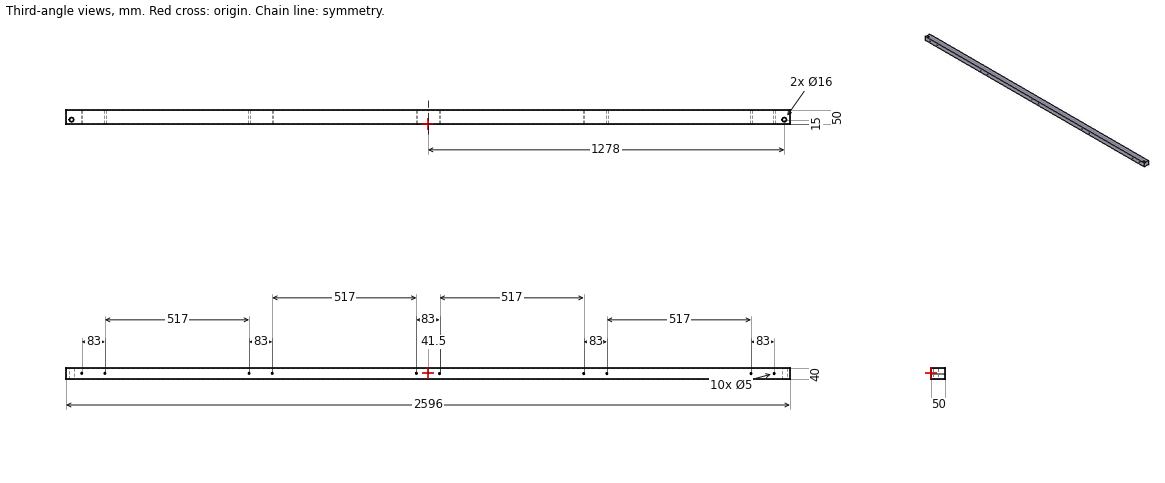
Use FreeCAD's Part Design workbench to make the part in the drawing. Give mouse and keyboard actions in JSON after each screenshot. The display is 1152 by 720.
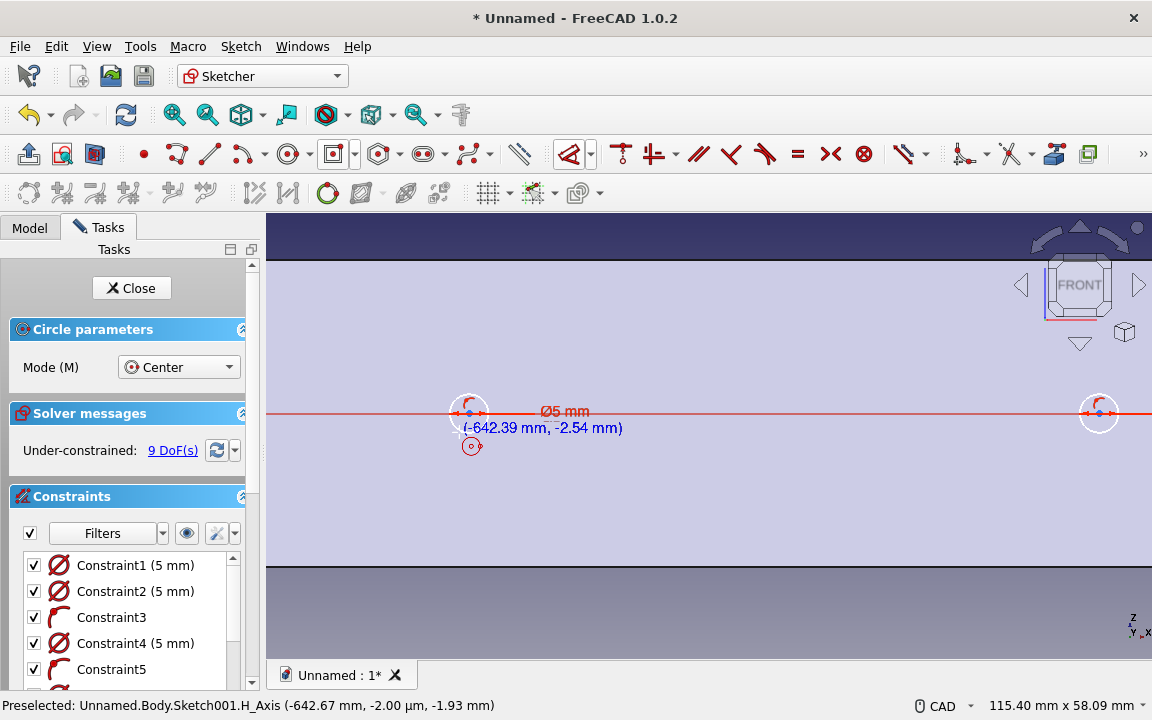
{"action": "scroll", "coordinate": [476, 437], "scroll_direction": "down", "scroll_amount": 17}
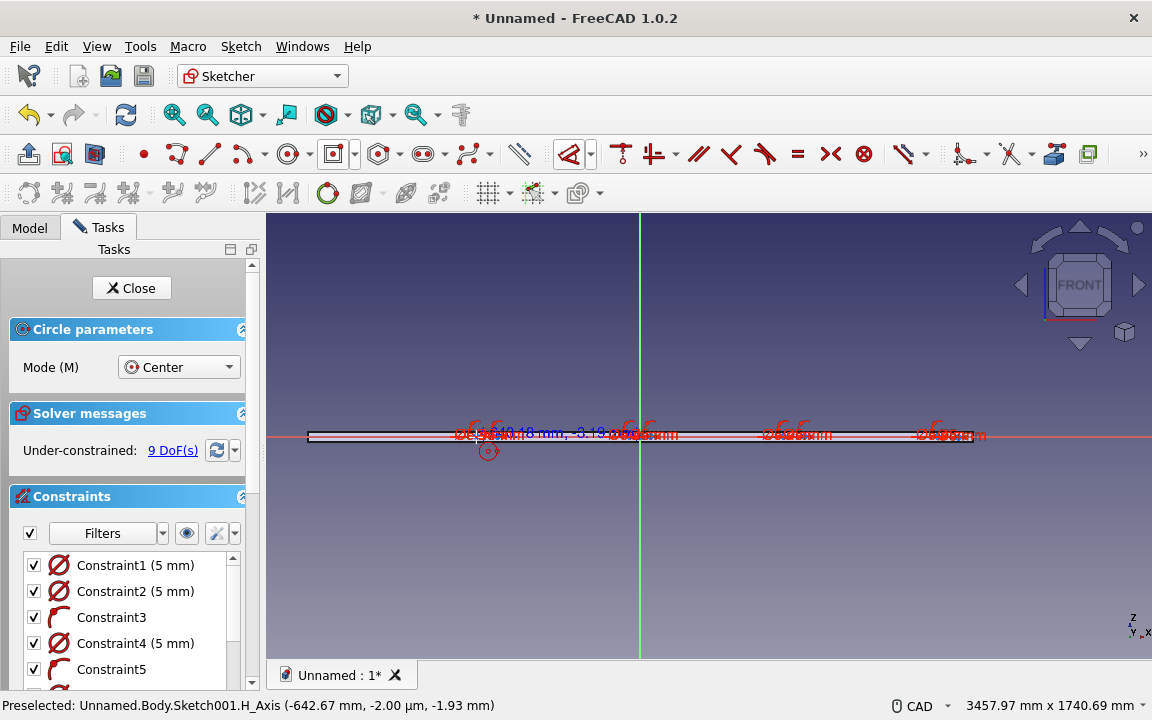
{"action": "scroll", "coordinate": [343, 437], "scroll_direction": "up", "scroll_amount": 18}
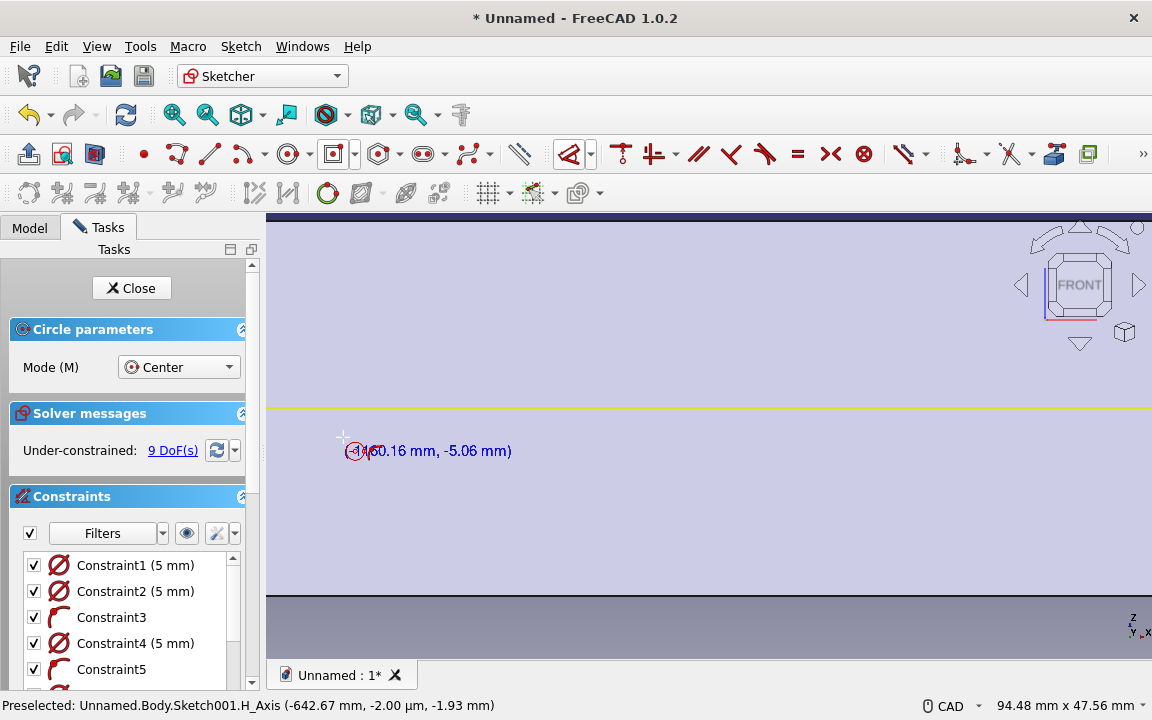
{"action": "scroll", "coordinate": [343, 437], "scroll_direction": "down", "scroll_amount": 18}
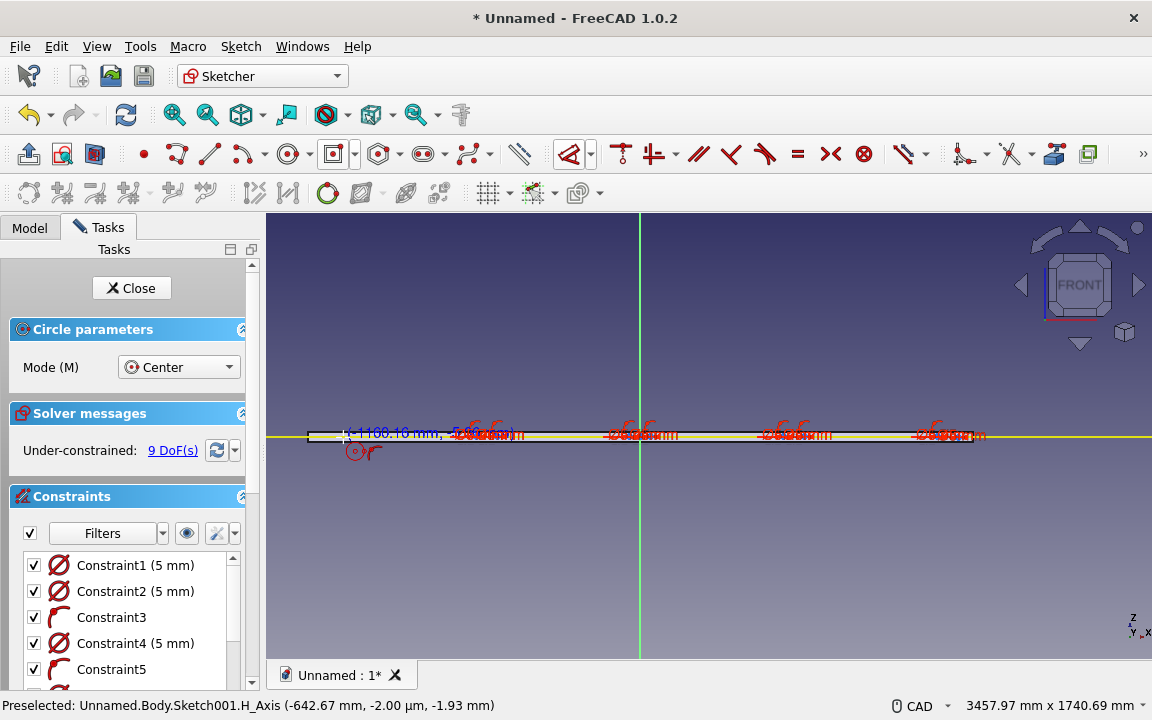
{"action": "left_click", "coordinate": [343, 437]}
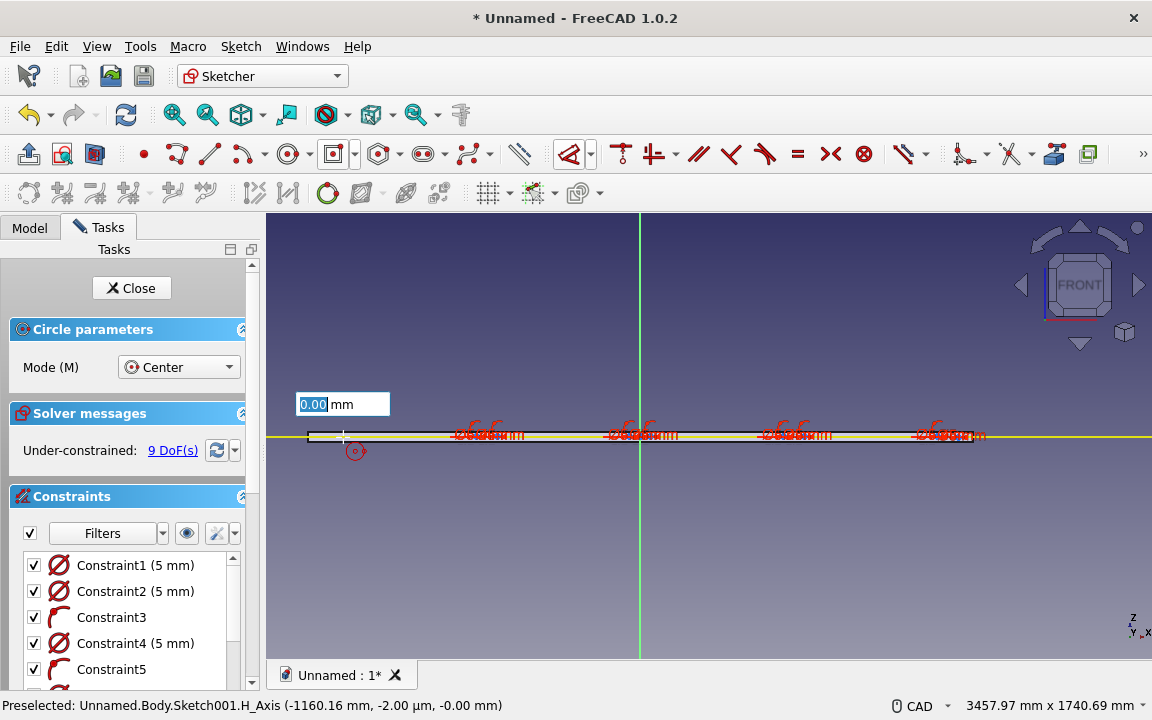
{"action": "scroll", "coordinate": [343, 437], "scroll_direction": "up", "scroll_amount": 17}
{"action": "mouse_move", "coordinate": [347, 432]}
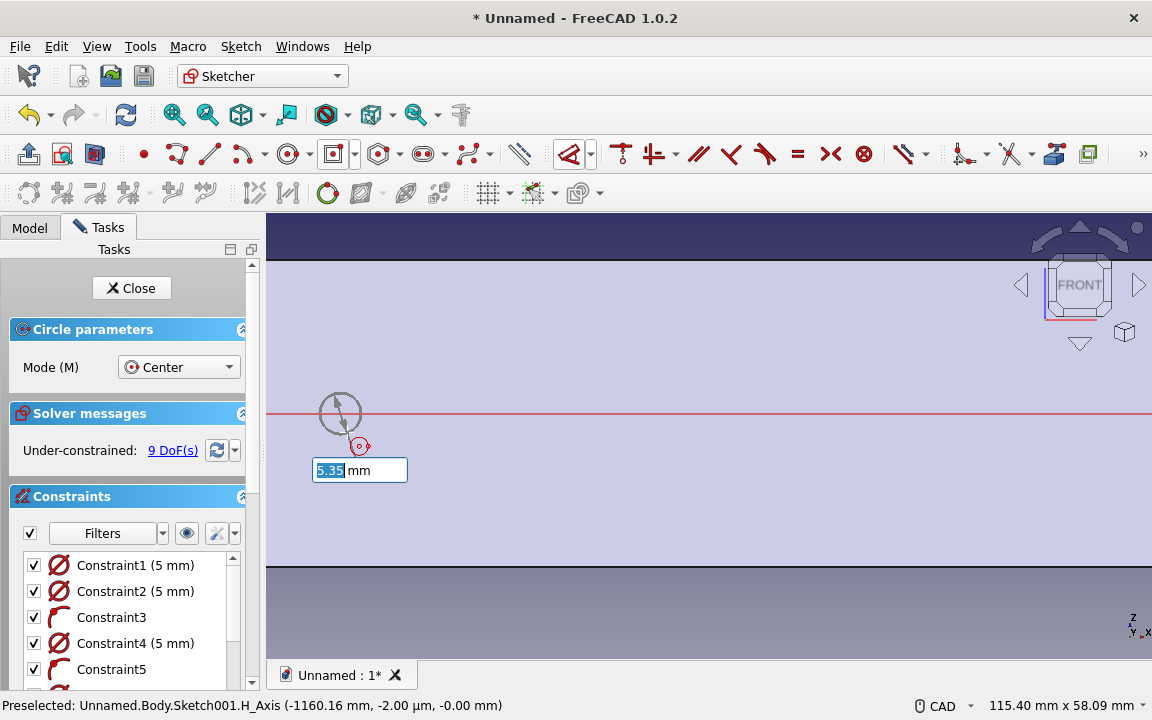
{"action": "type", "text": "5"}
{"action": "key", "text": "Return"}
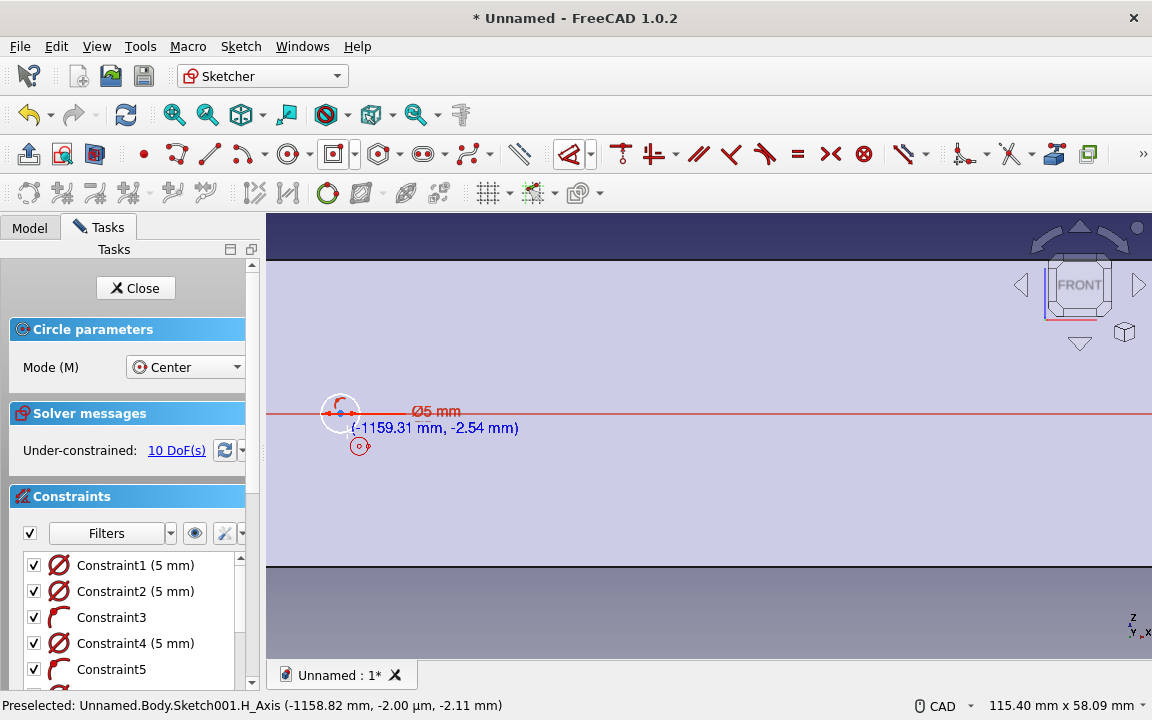
{"action": "scroll", "coordinate": [343, 437], "scroll_direction": "down", "scroll_amount": 17}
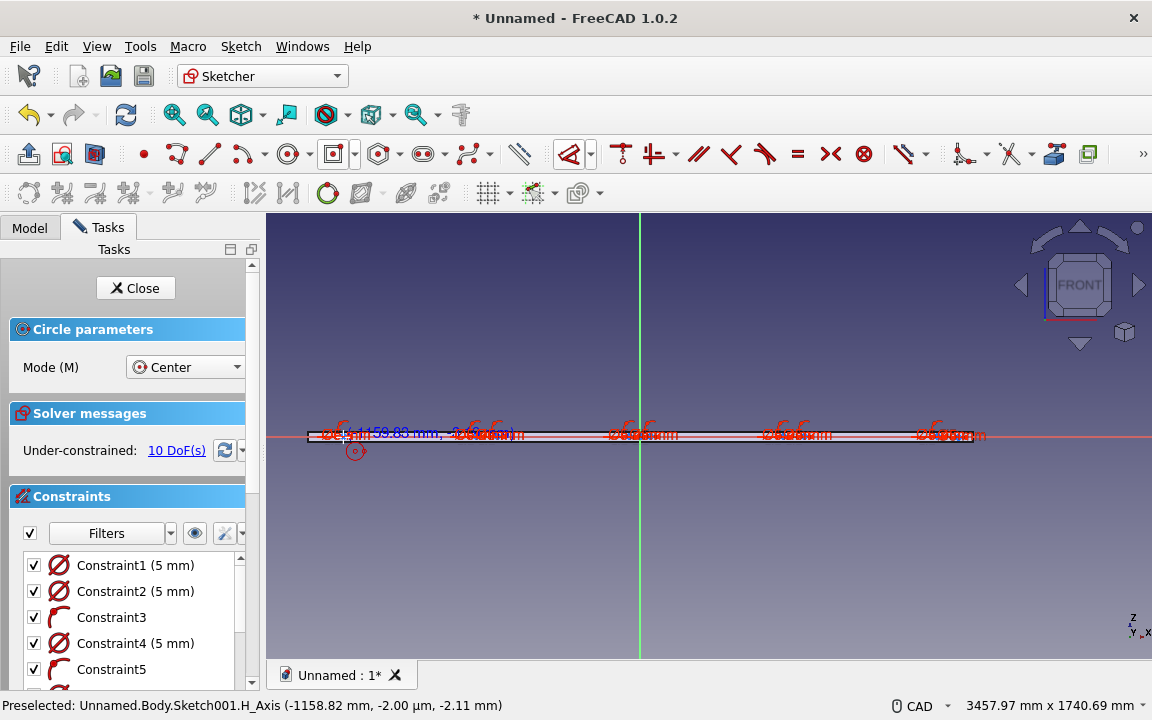
{"action": "scroll", "coordinate": [322, 437], "scroll_direction": "up", "scroll_amount": 18}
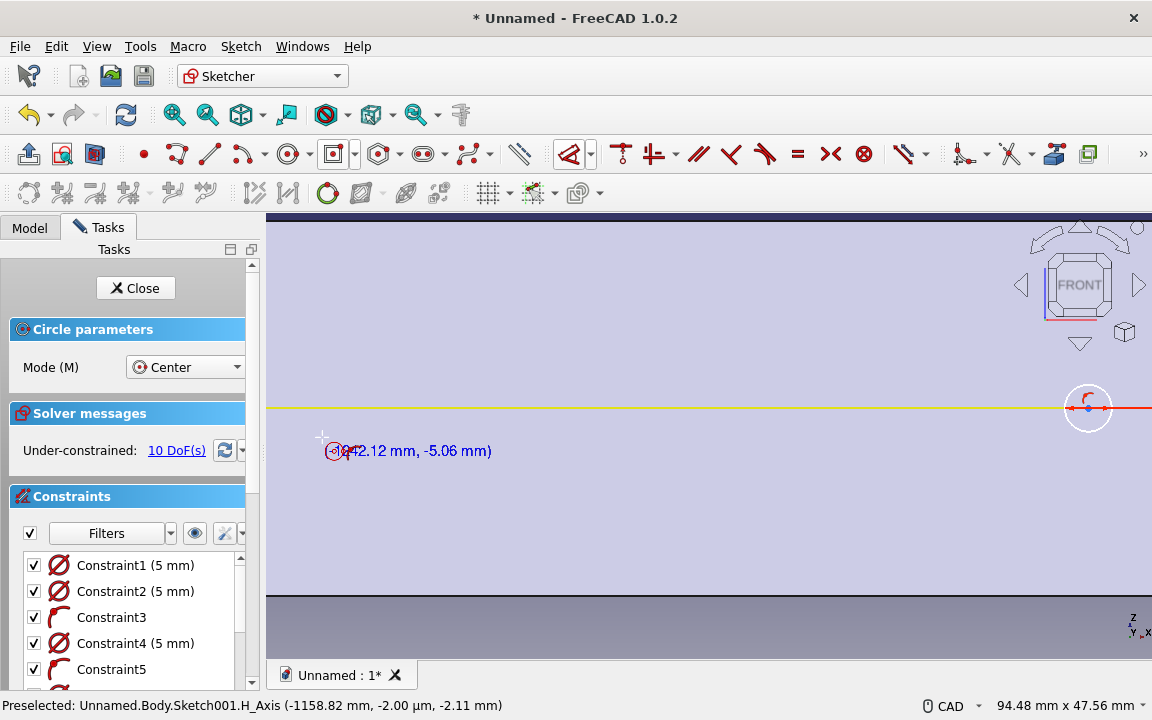
{"action": "scroll", "coordinate": [322, 437], "scroll_direction": "down", "scroll_amount": 18}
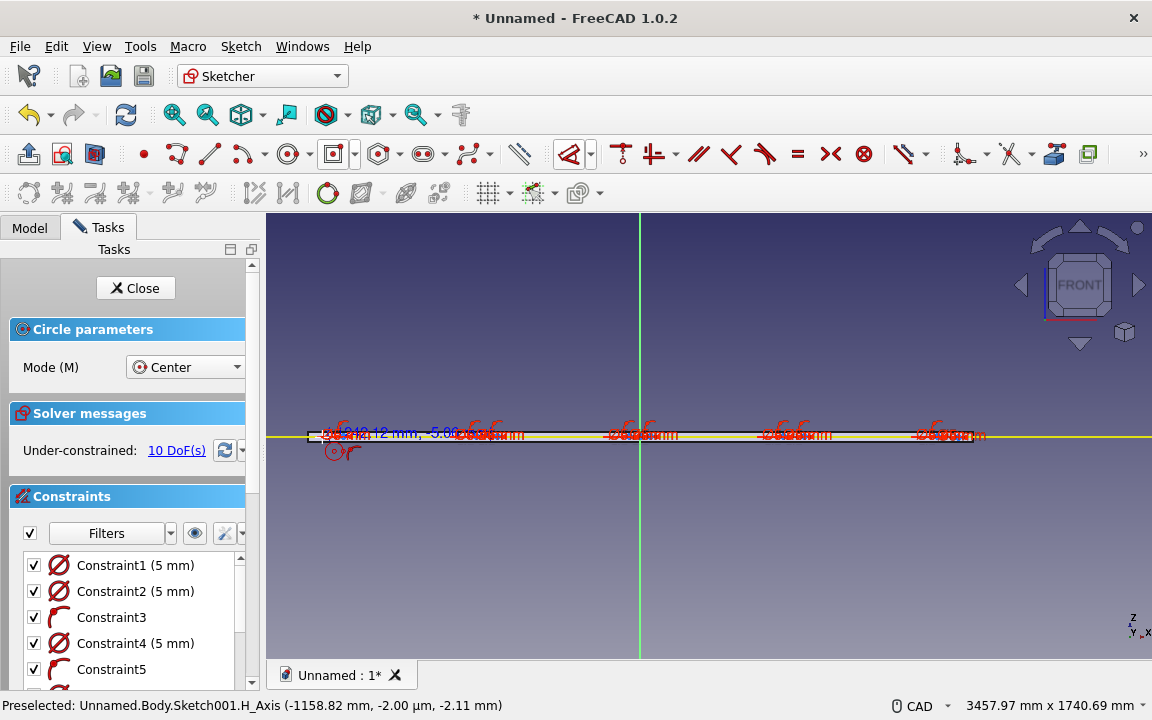
{"action": "left_click", "coordinate": [322, 437]}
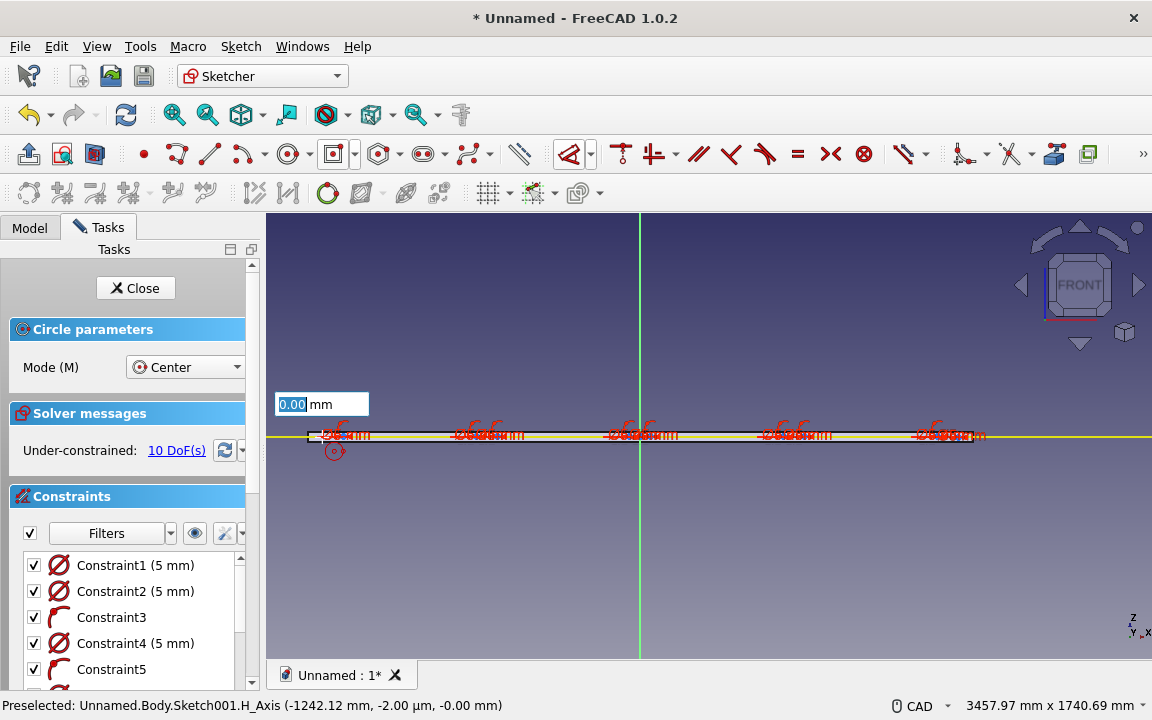
{"action": "scroll", "coordinate": [322, 437], "scroll_direction": "up", "scroll_amount": 17}
{"action": "mouse_move", "coordinate": [318, 432]}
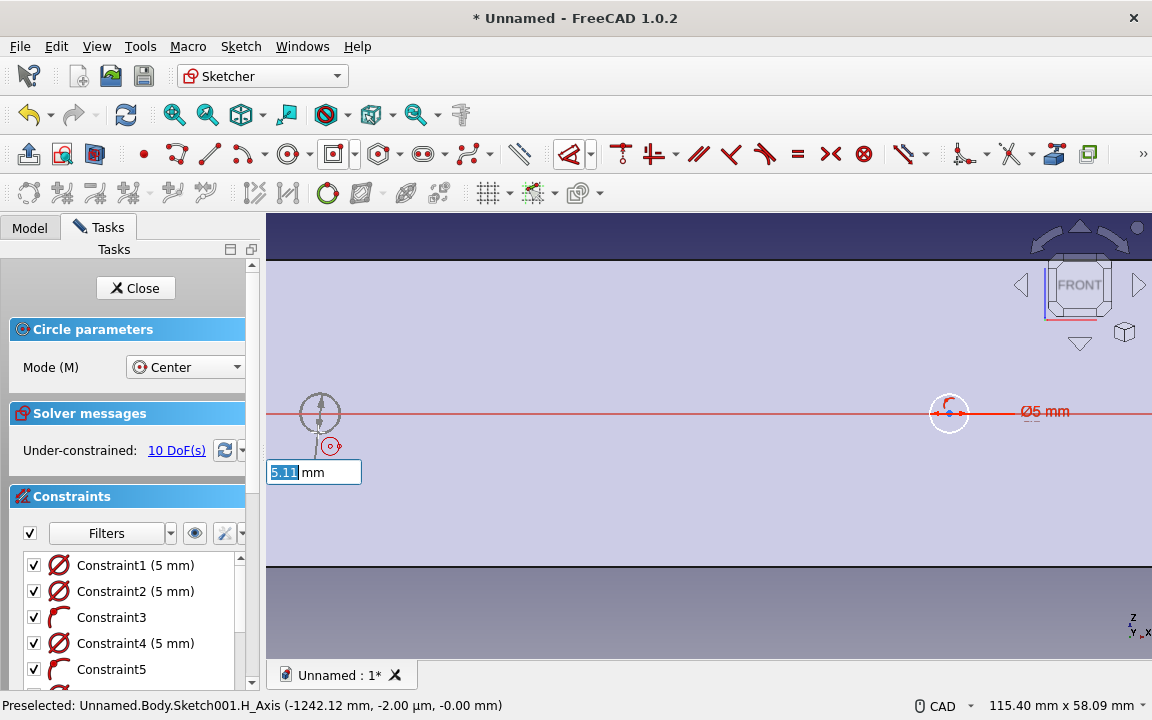
{"action": "type", "text": "5"}
{"action": "key", "text": "Return"}
{"action": "key", "text": "Escape"}